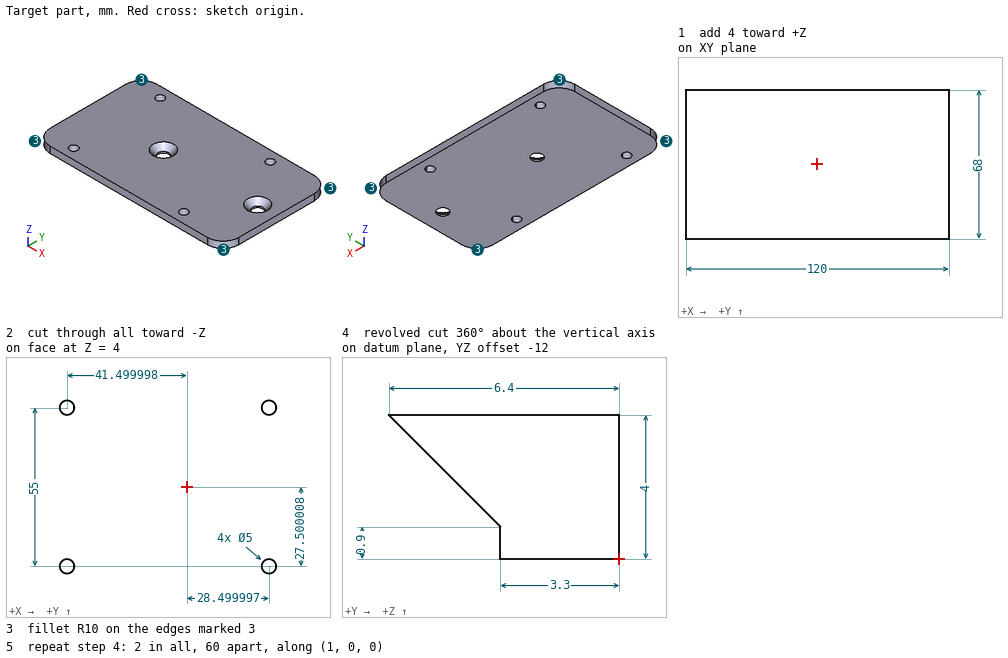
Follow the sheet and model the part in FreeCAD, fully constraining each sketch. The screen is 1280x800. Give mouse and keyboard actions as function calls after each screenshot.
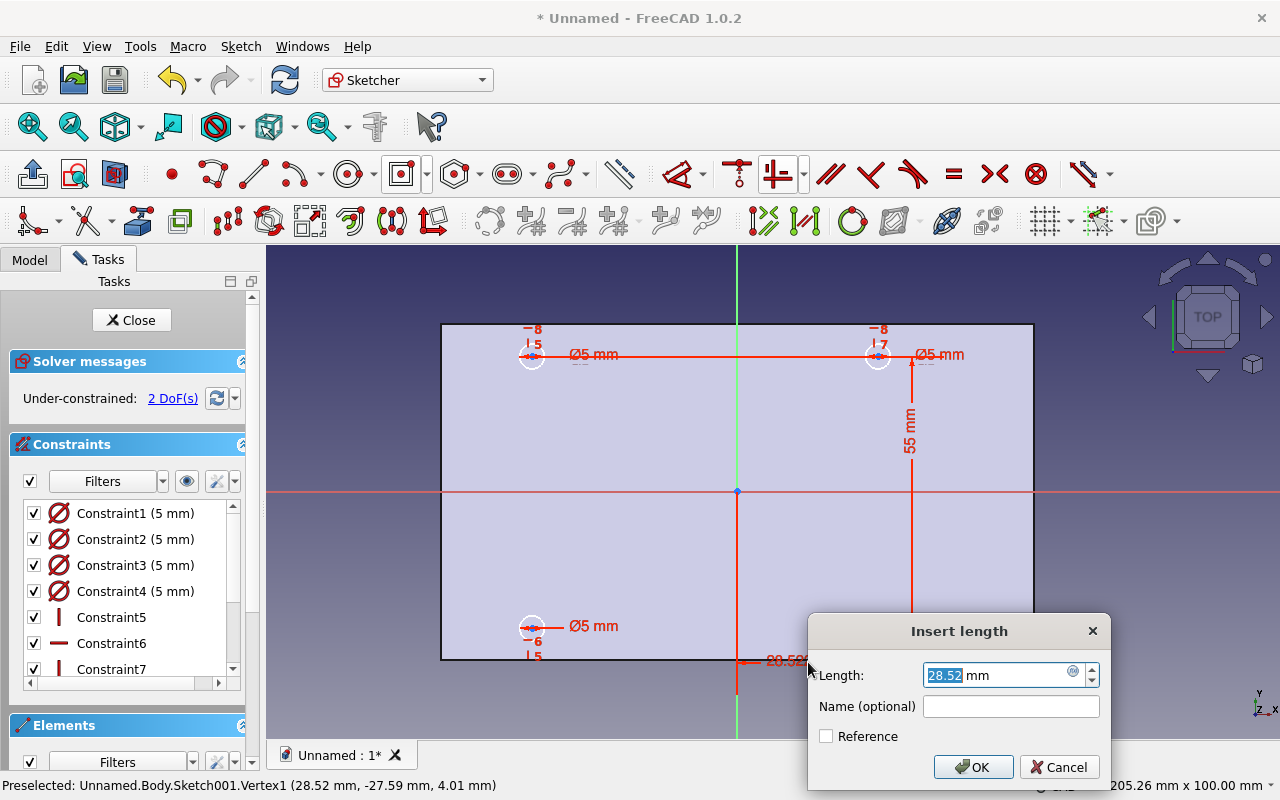
text(28.499997)
key(Return)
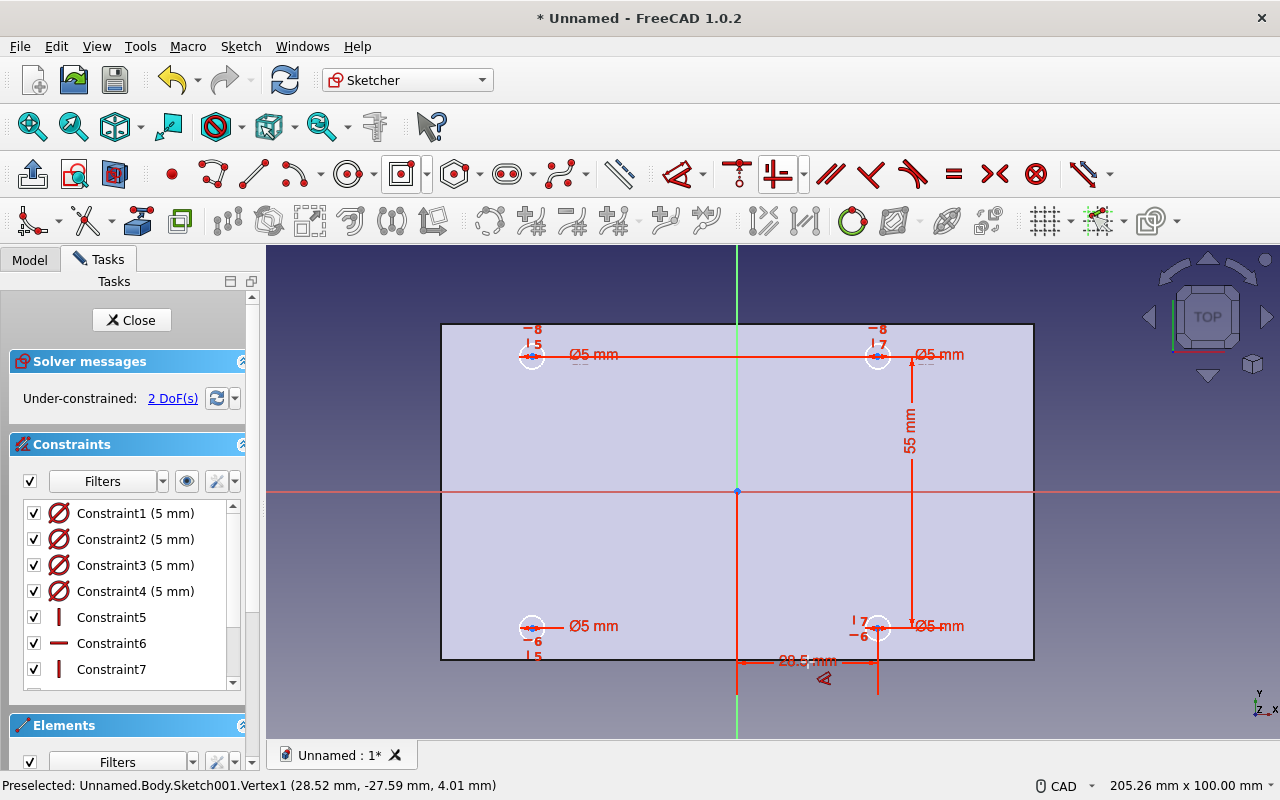
click(878, 628)
click(912, 560)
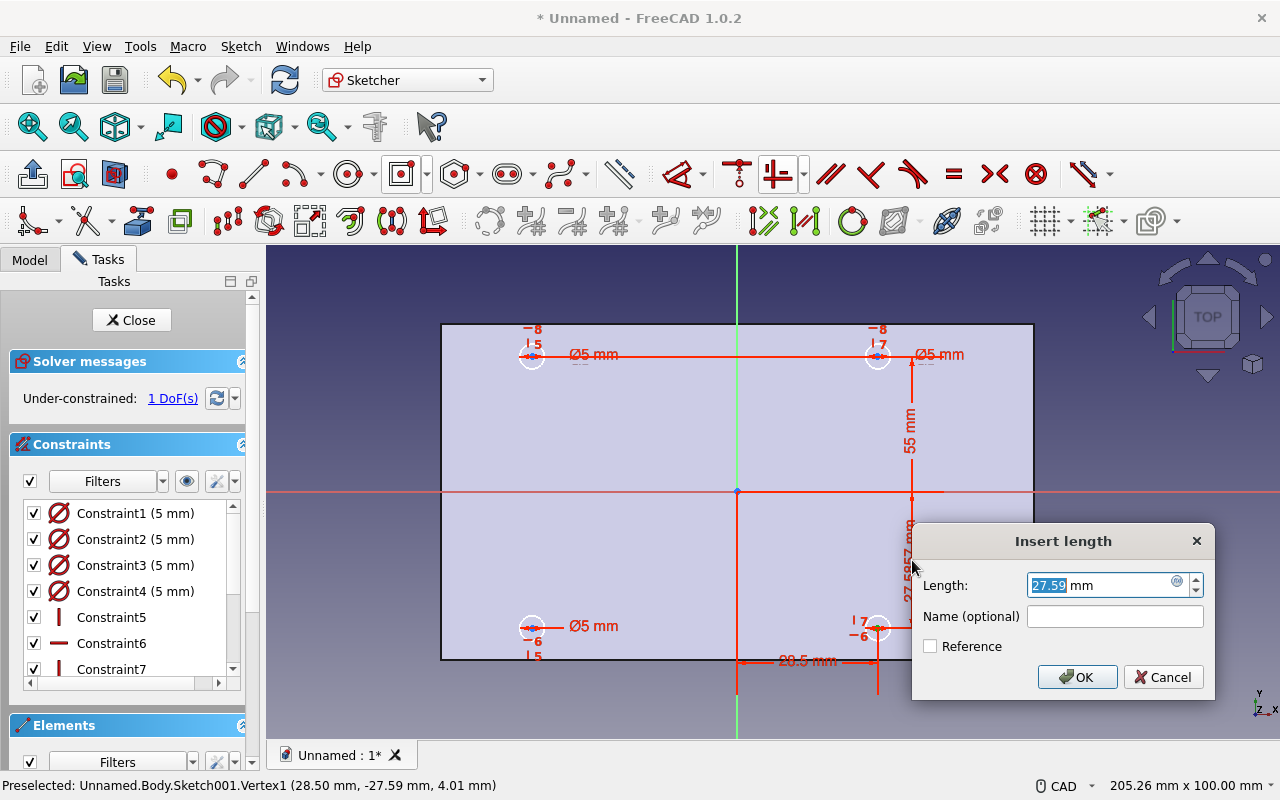
text(27.500008)
key(Return)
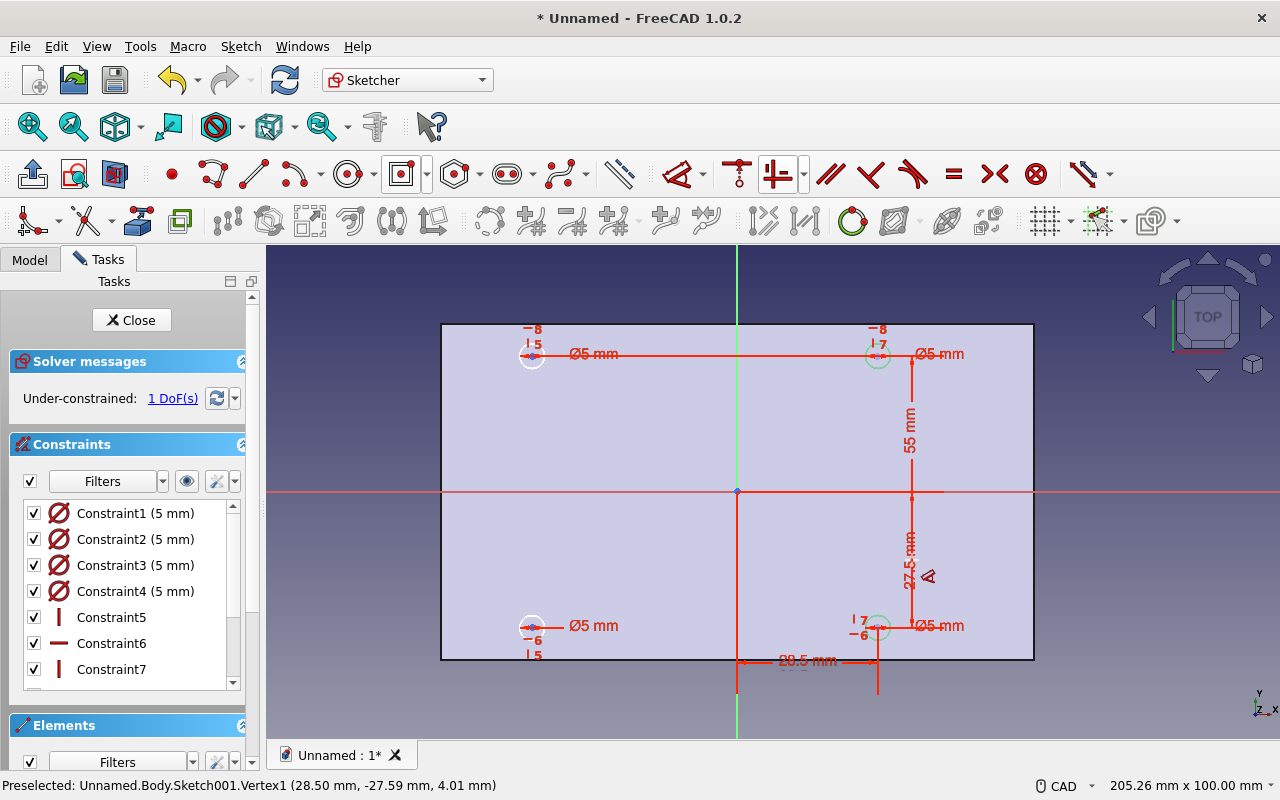
click(532, 356)
click(635, 322)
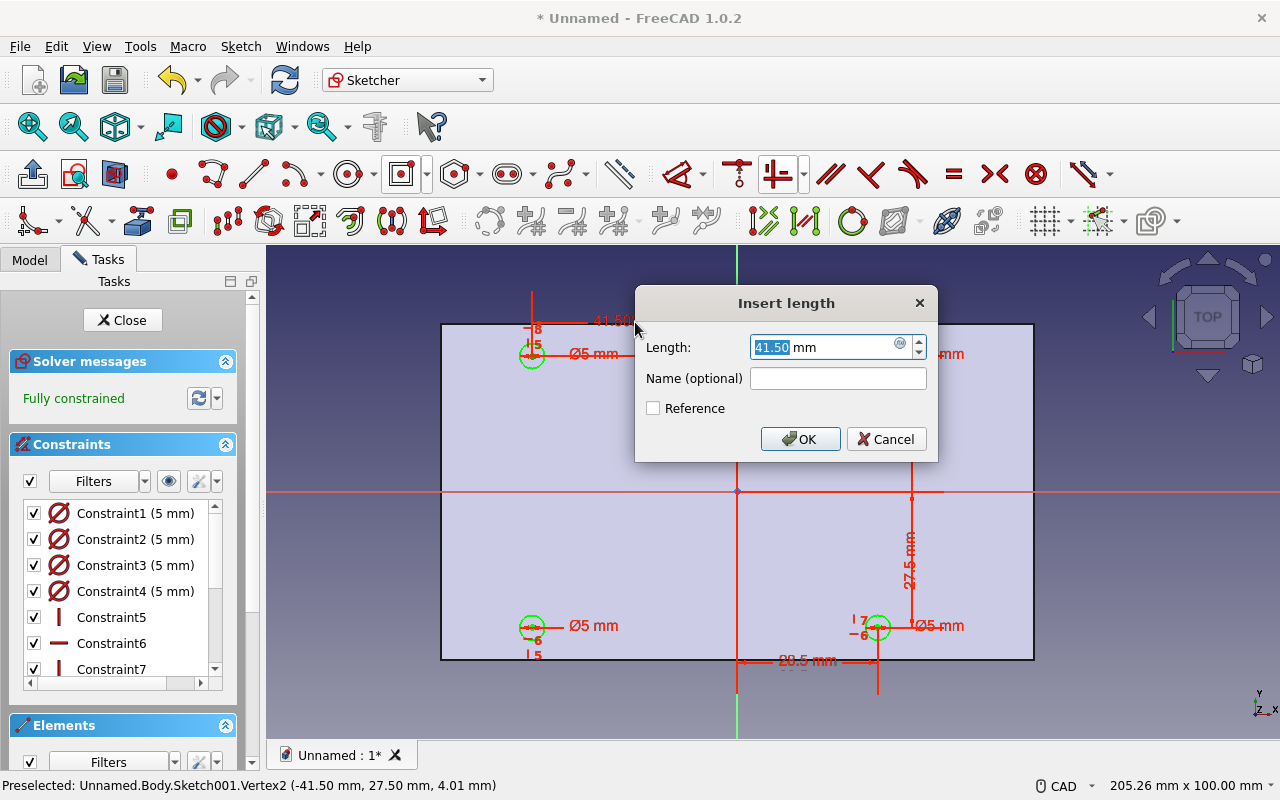
text(41.499998)
key(Return)
key(Escape)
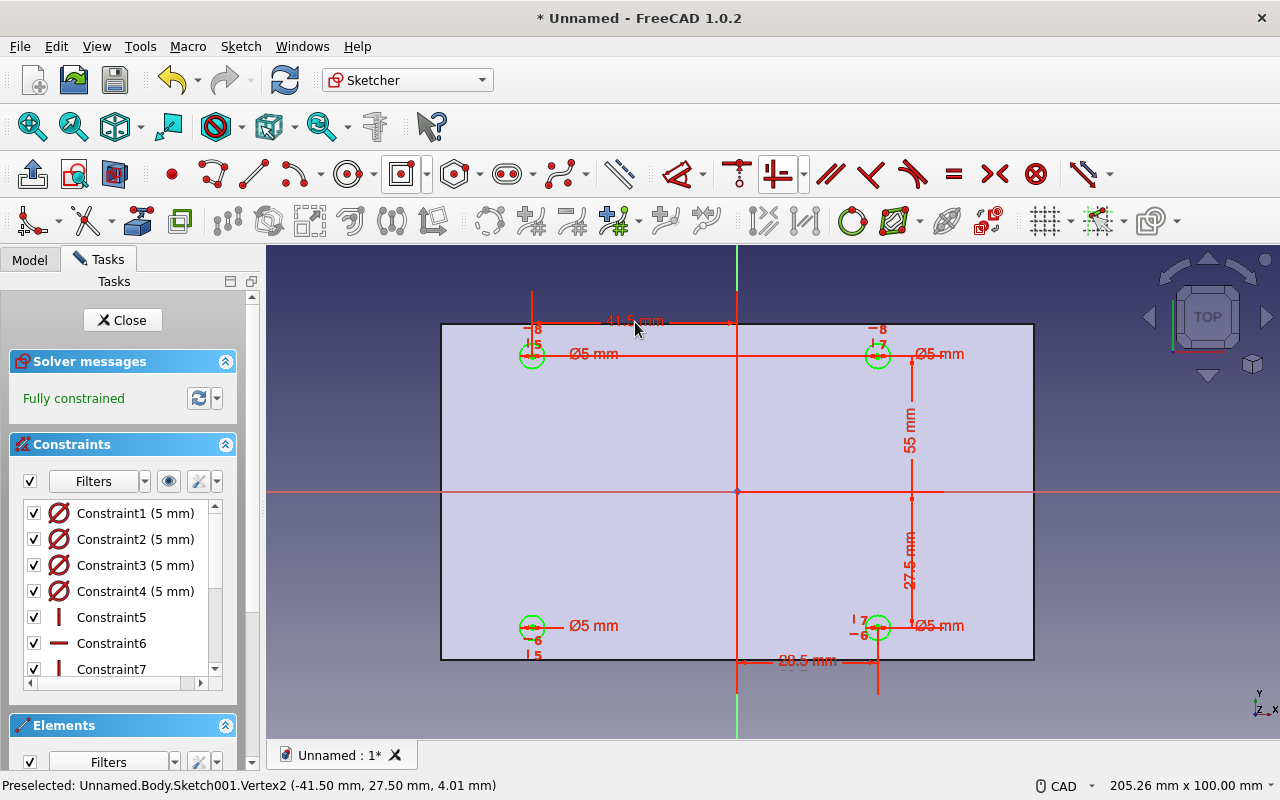
click(123, 320)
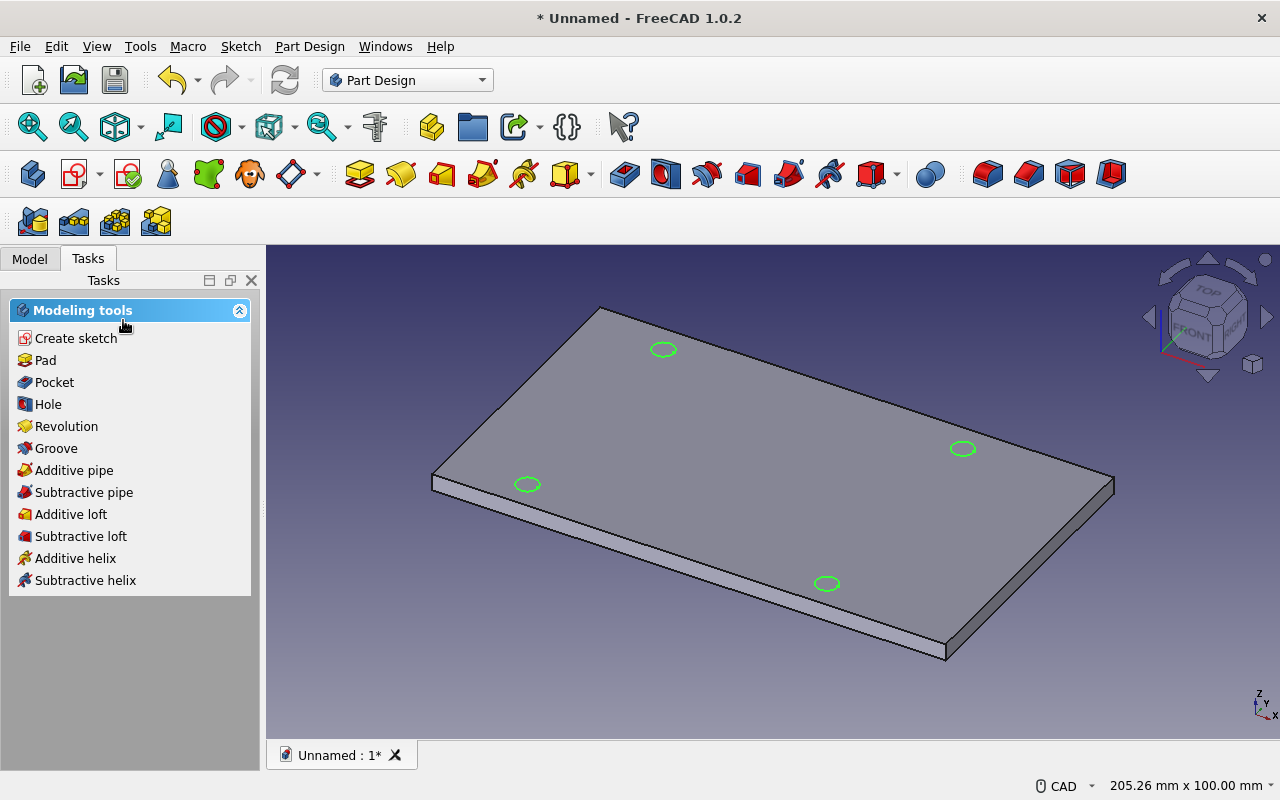
click(625, 174)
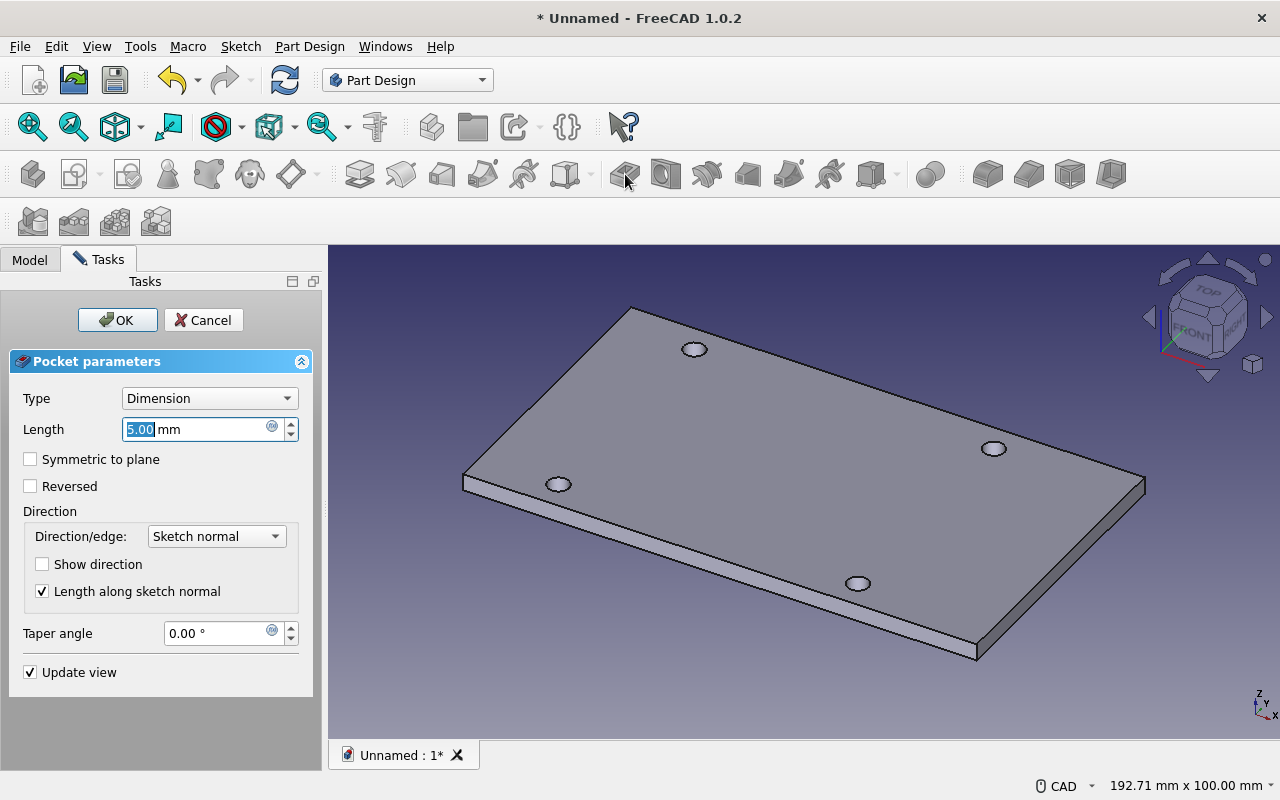
click(210, 398)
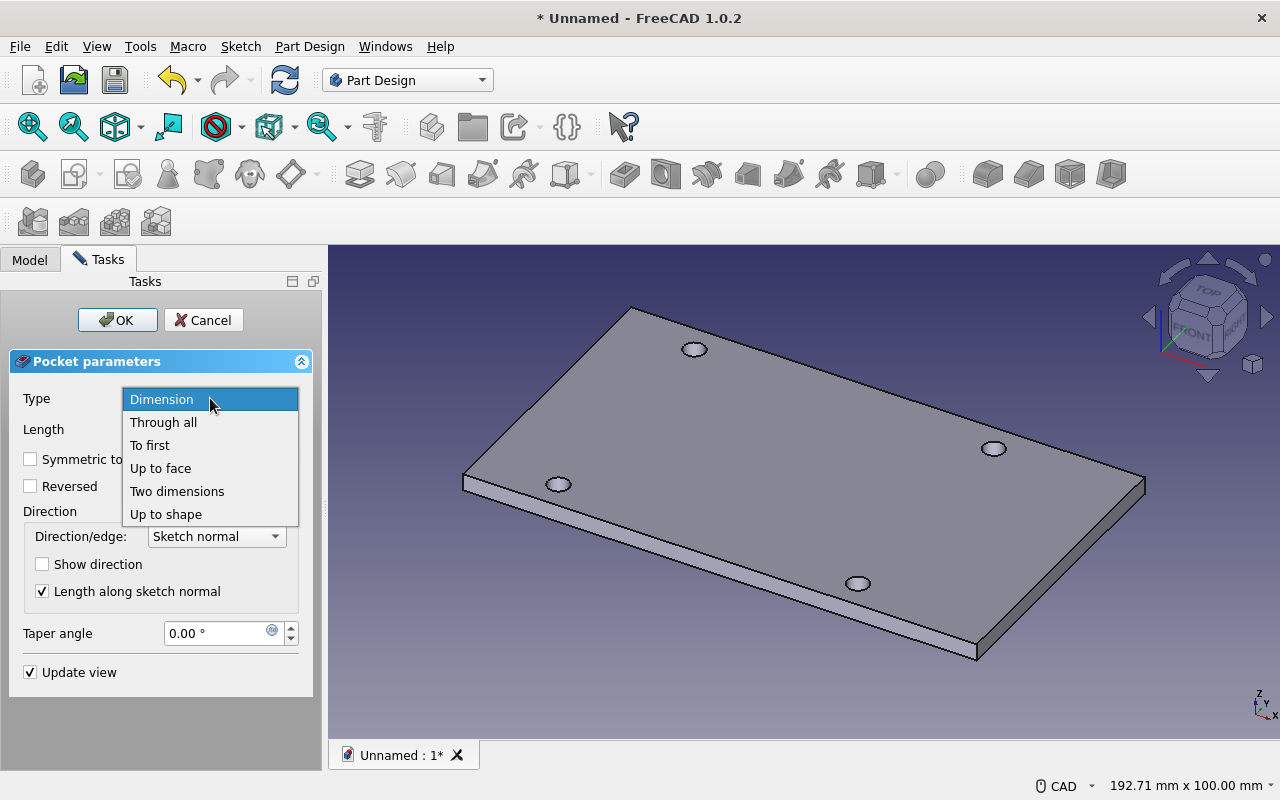
click(208, 422)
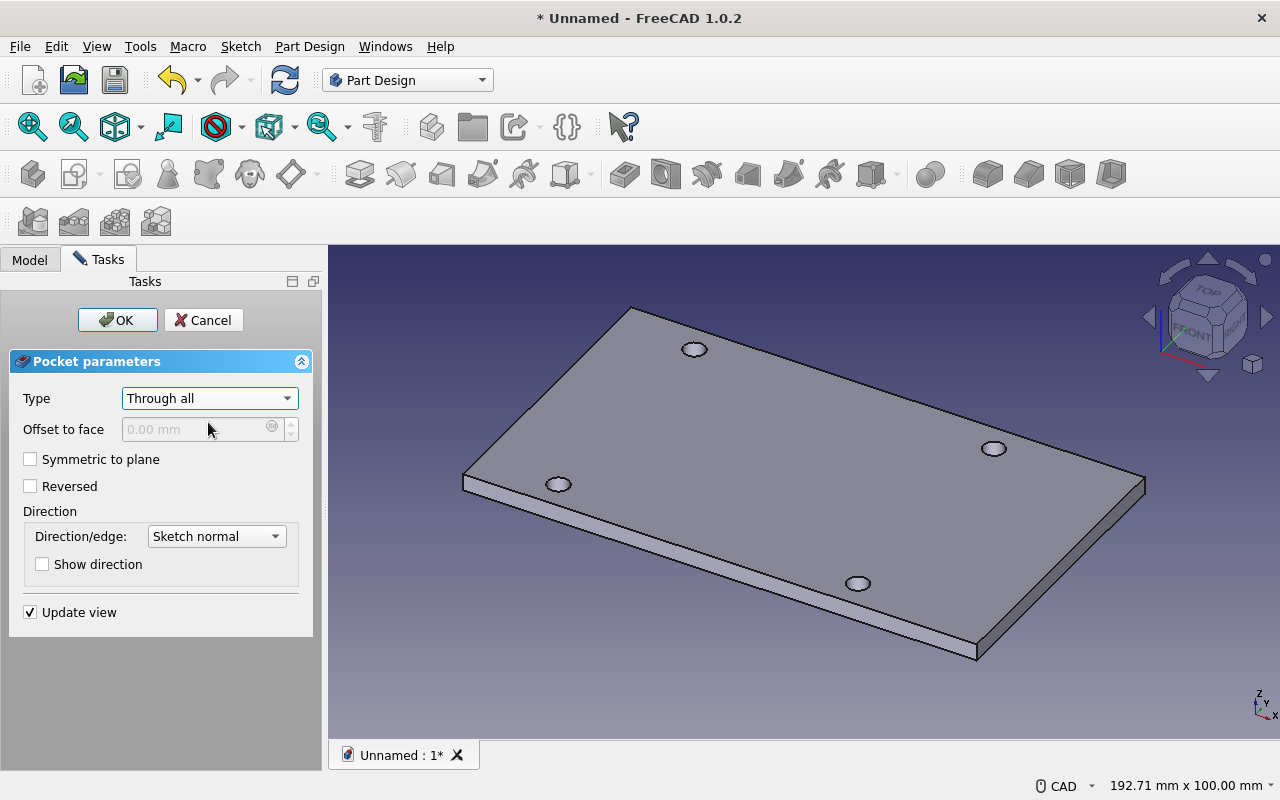
click(118, 320)